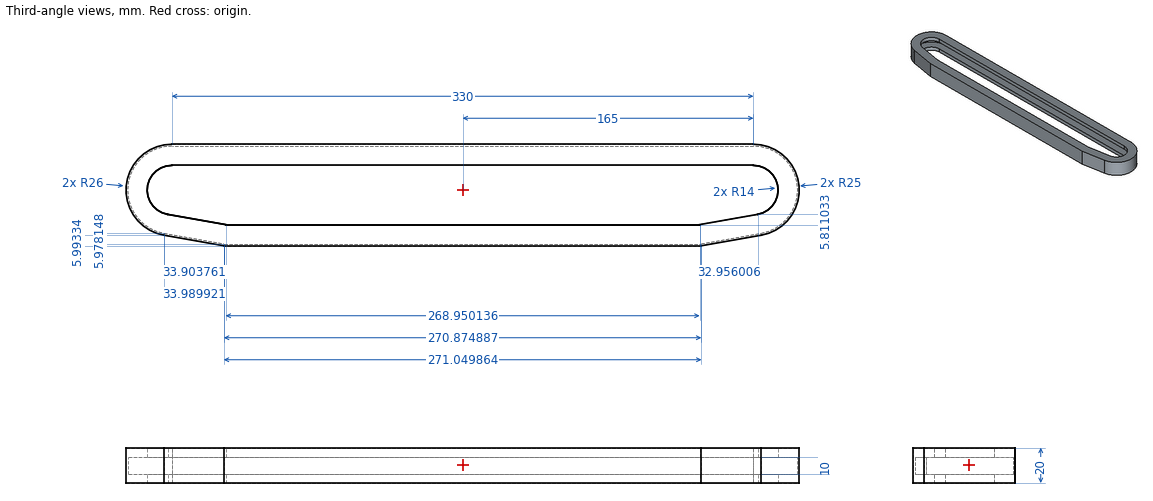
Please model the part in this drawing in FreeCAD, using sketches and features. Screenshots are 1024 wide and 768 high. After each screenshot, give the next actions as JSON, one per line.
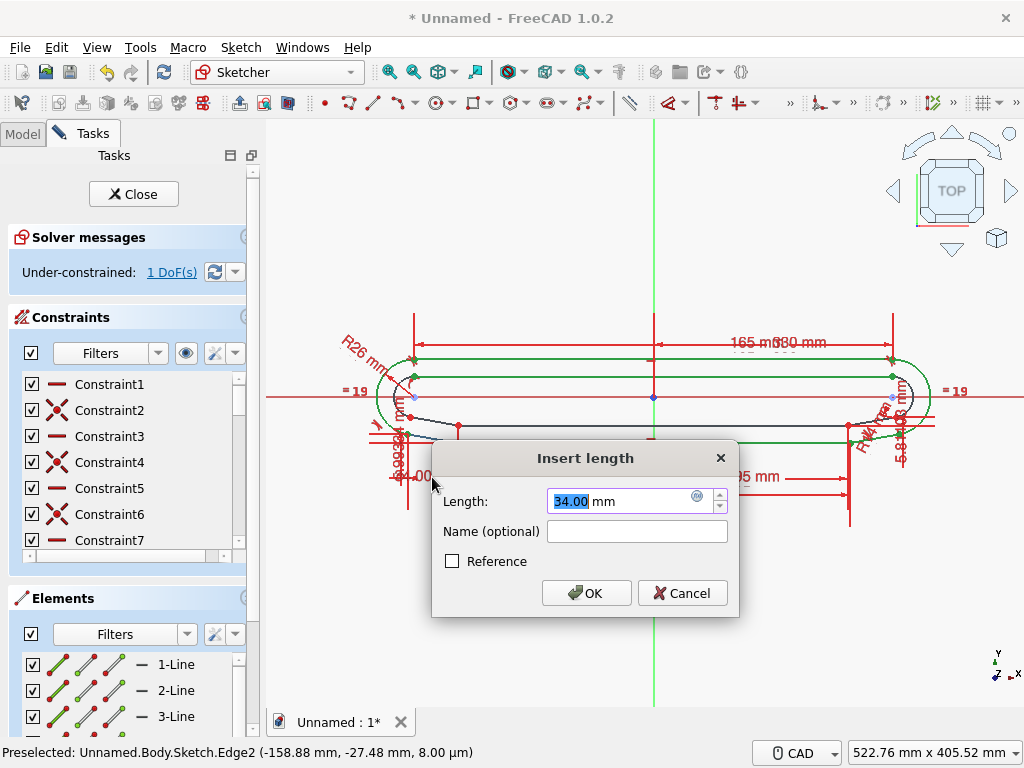
{"action": "type", "text": "33.989921"}
{"action": "key", "text": "Return"}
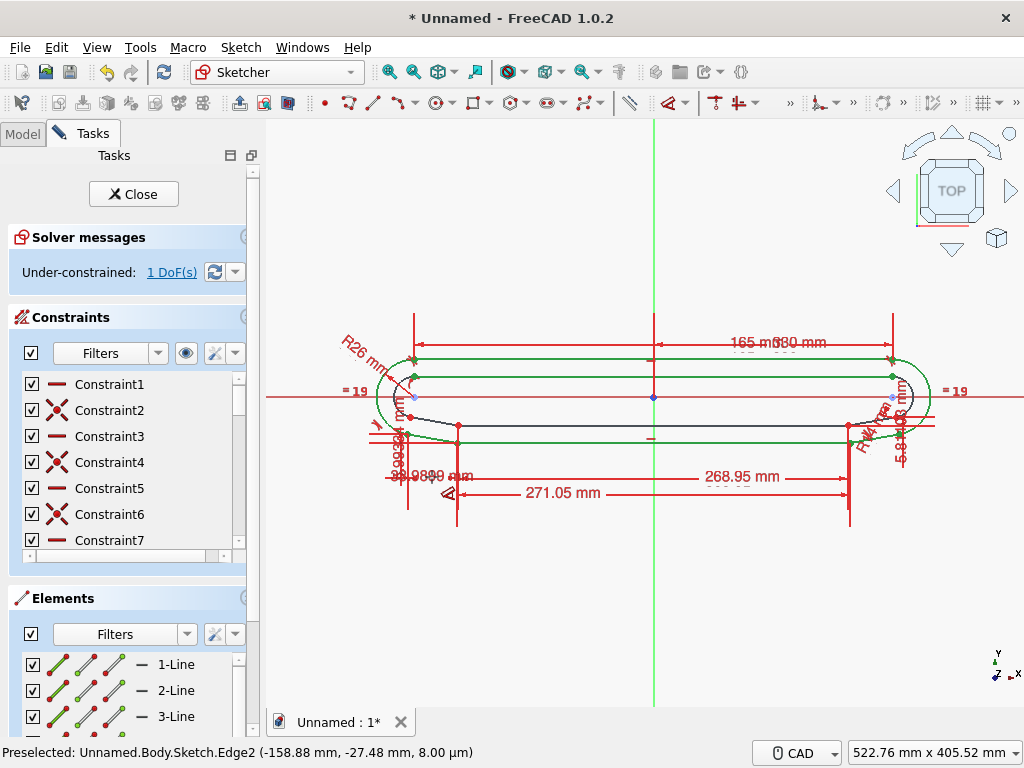
{"action": "scroll", "coordinate": [858, 424], "scroll_direction": "up", "scroll_amount": 2}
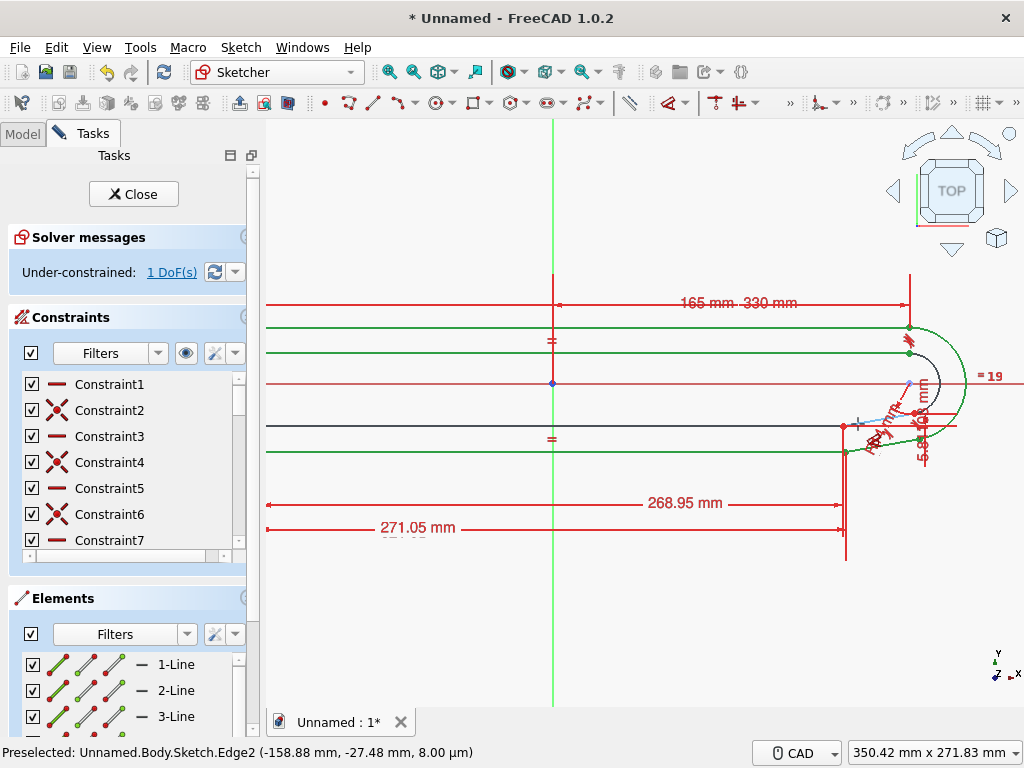
{"action": "left_click", "coordinate": [858, 424]}
{"action": "left_click", "coordinate": [851, 484]}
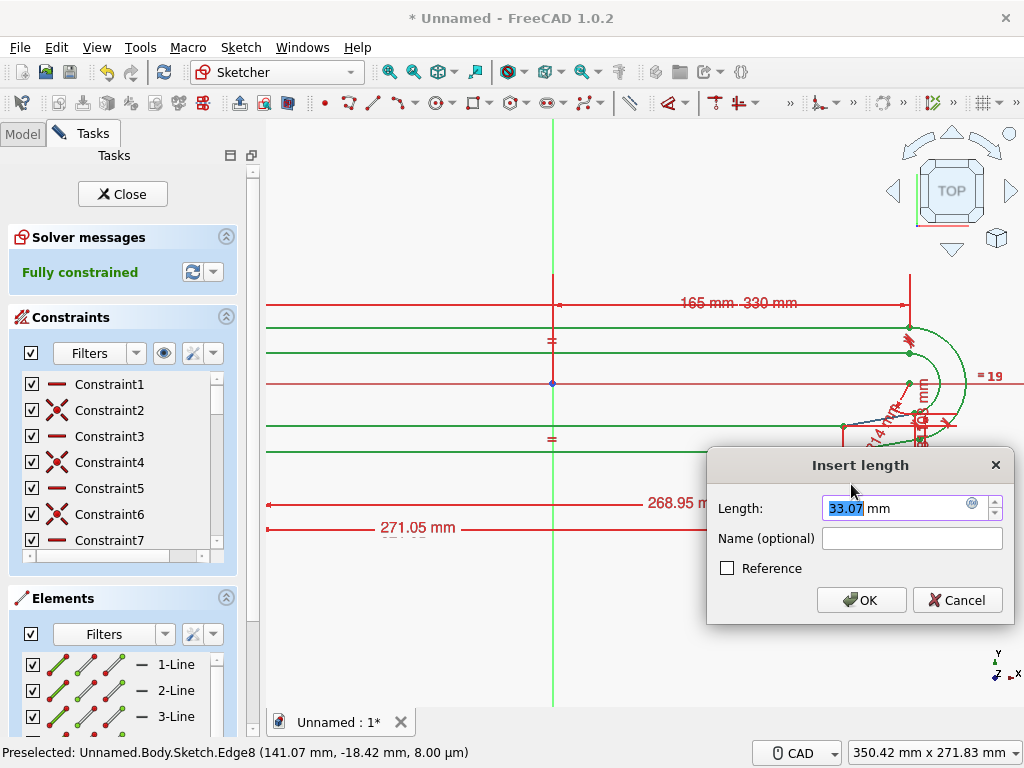
{"action": "type", "text": "32.956006"}
{"action": "key", "text": "Return"}
{"action": "key", "text": "Escape"}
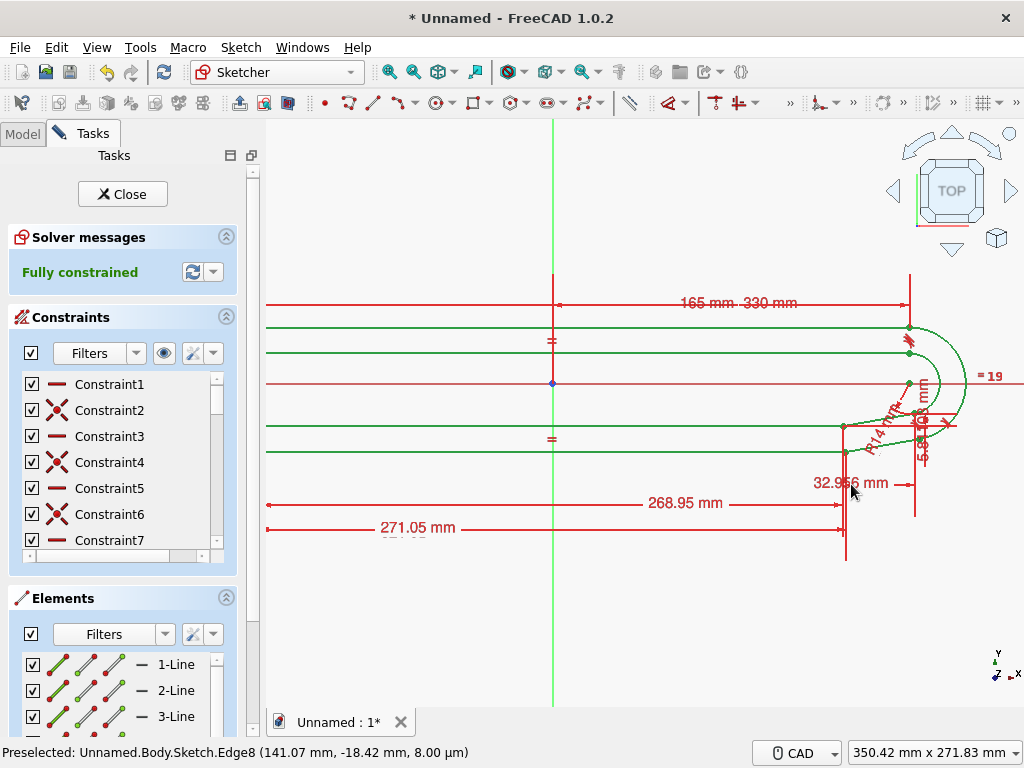
{"action": "left_click", "coordinate": [123, 194]}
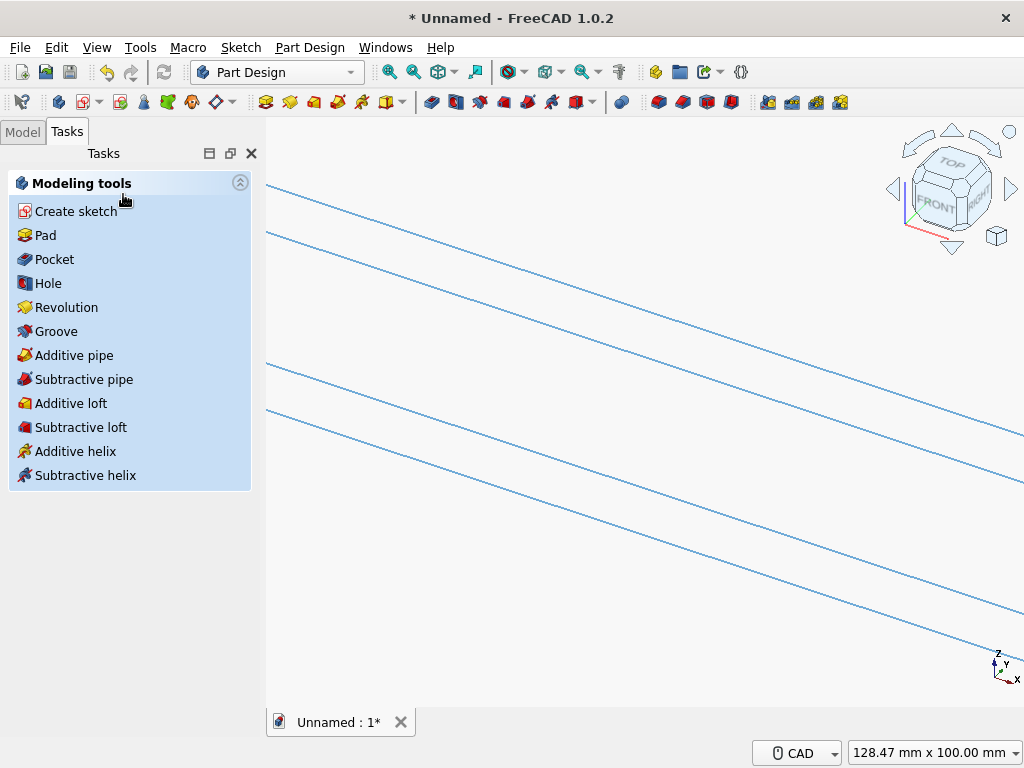
{"action": "left_click", "coordinate": [266, 102]}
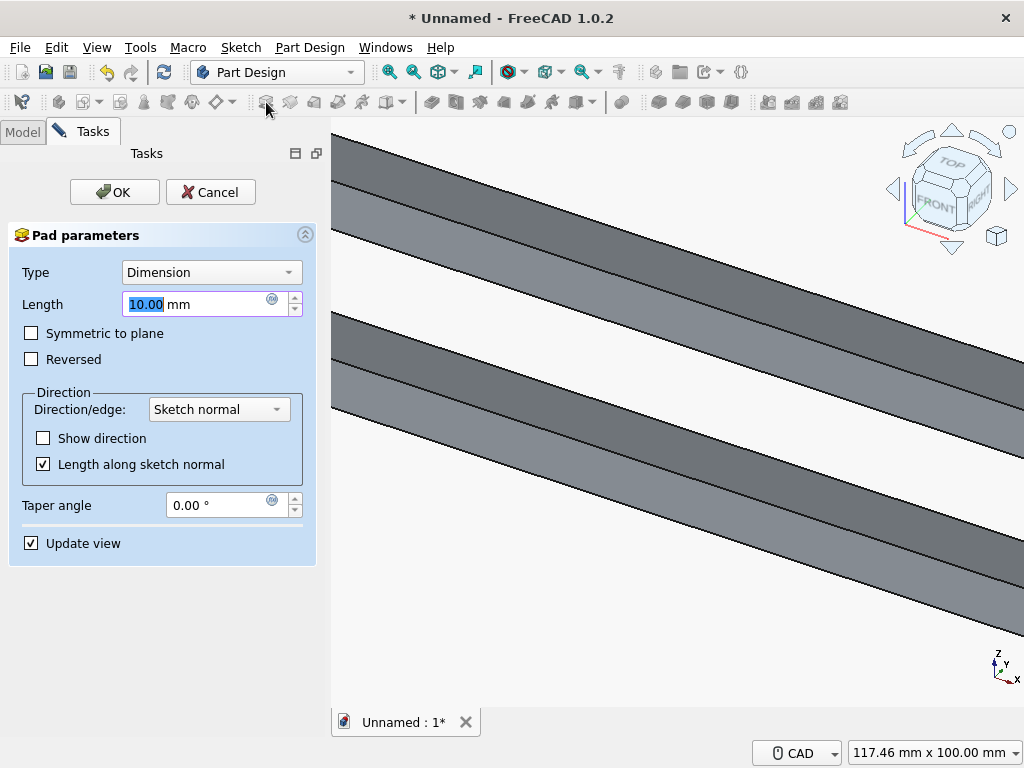
{"action": "type", "text": "20"}
{"action": "key", "text": "Tab"}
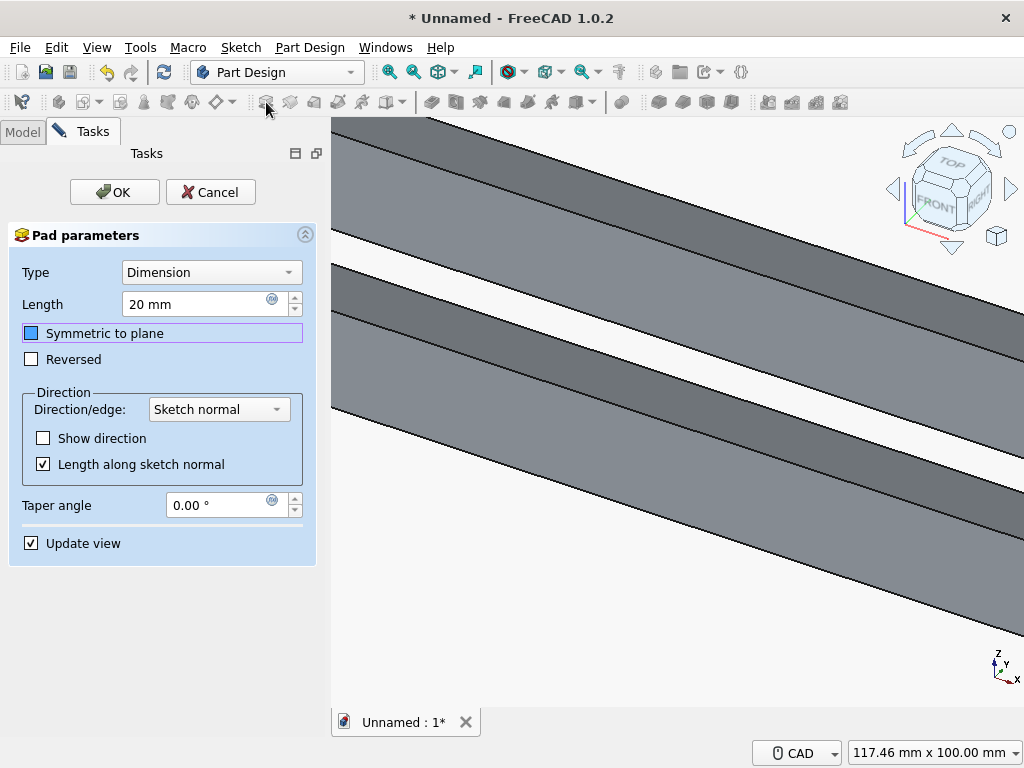
{"action": "left_click", "coordinate": [30, 333]}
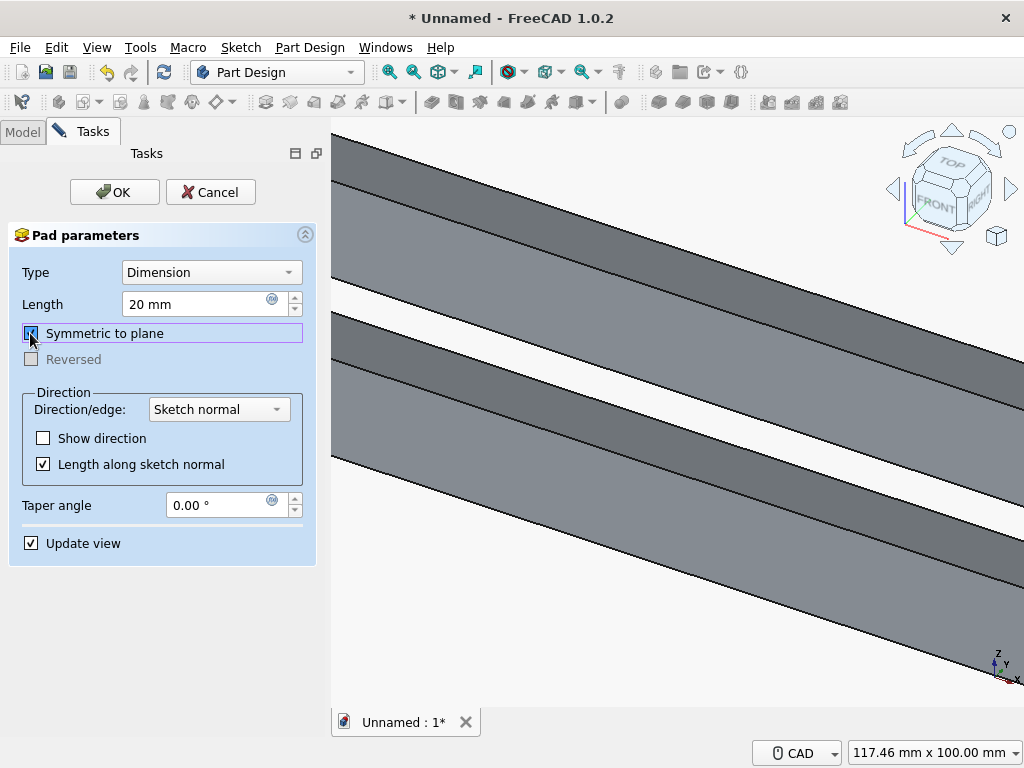
{"action": "left_click", "coordinate": [115, 192]}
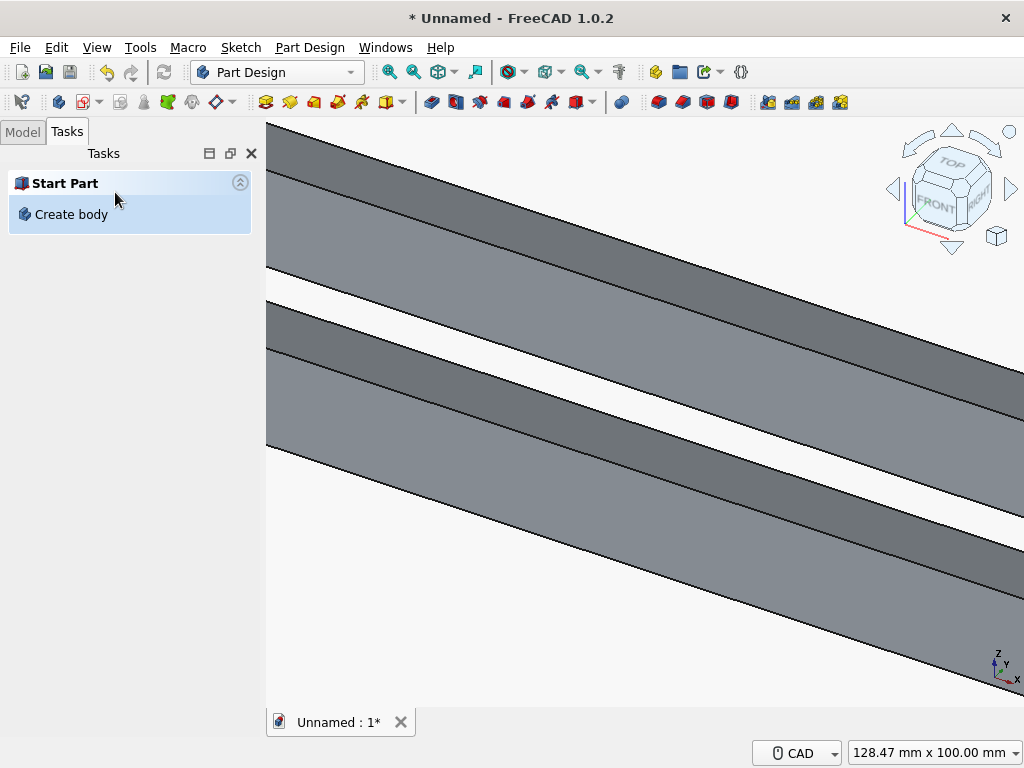
{"action": "left_click", "coordinate": [390, 72]}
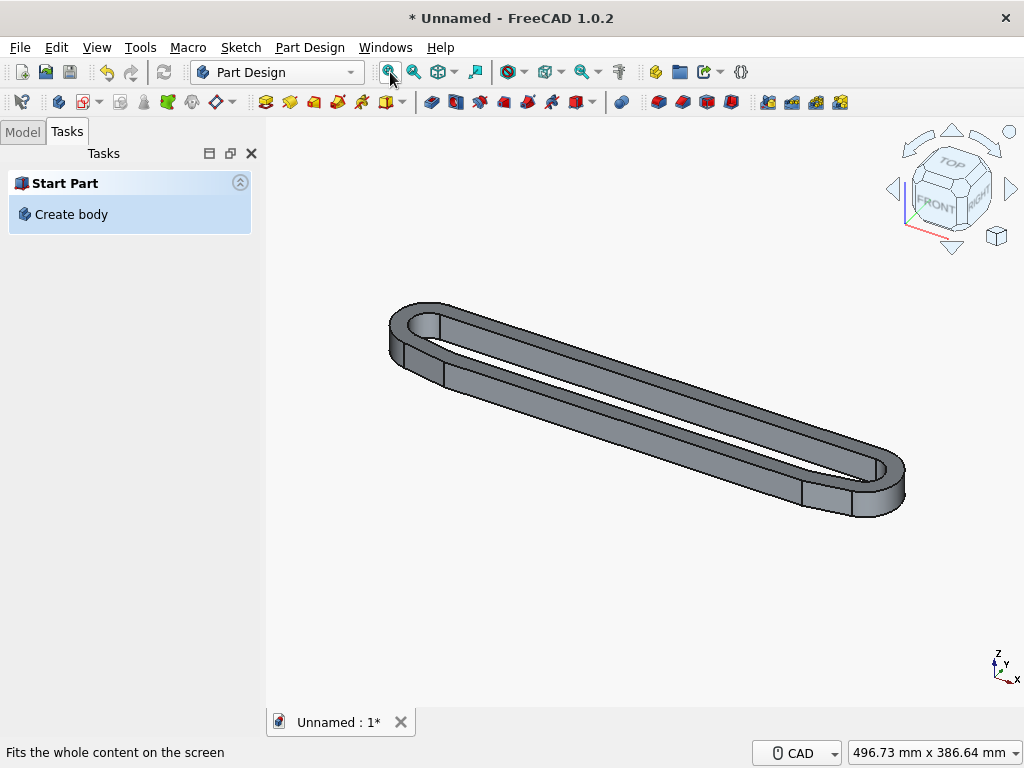
{"action": "left_click", "coordinate": [84, 102]}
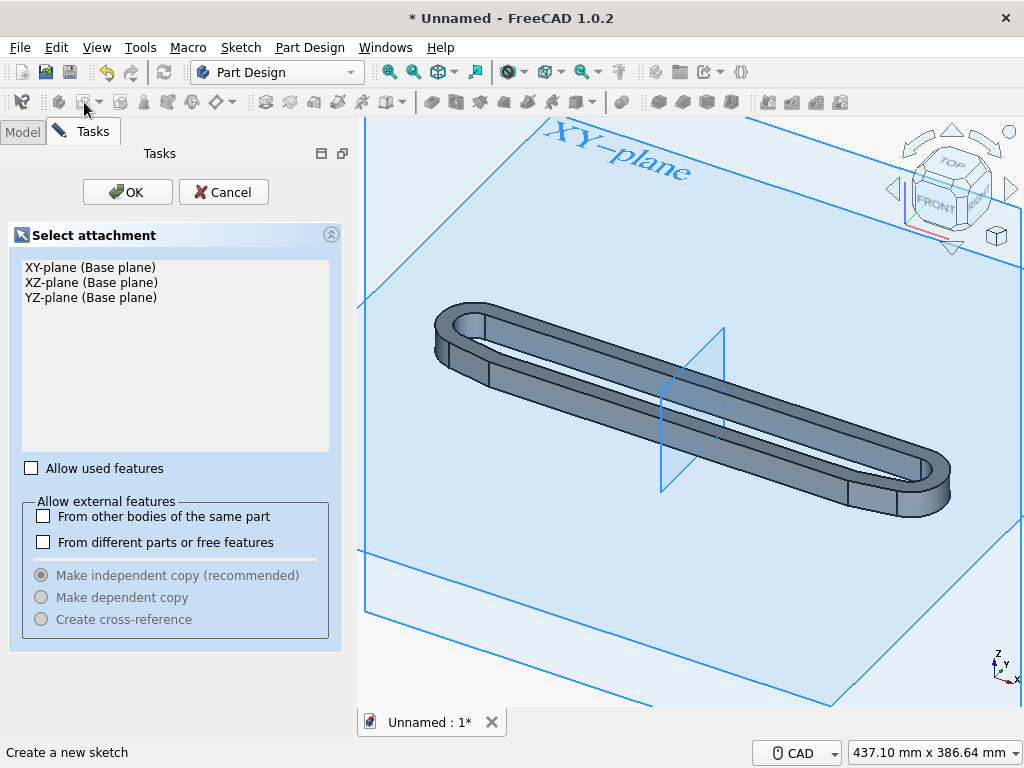
{"action": "left_click", "coordinate": [82, 268]}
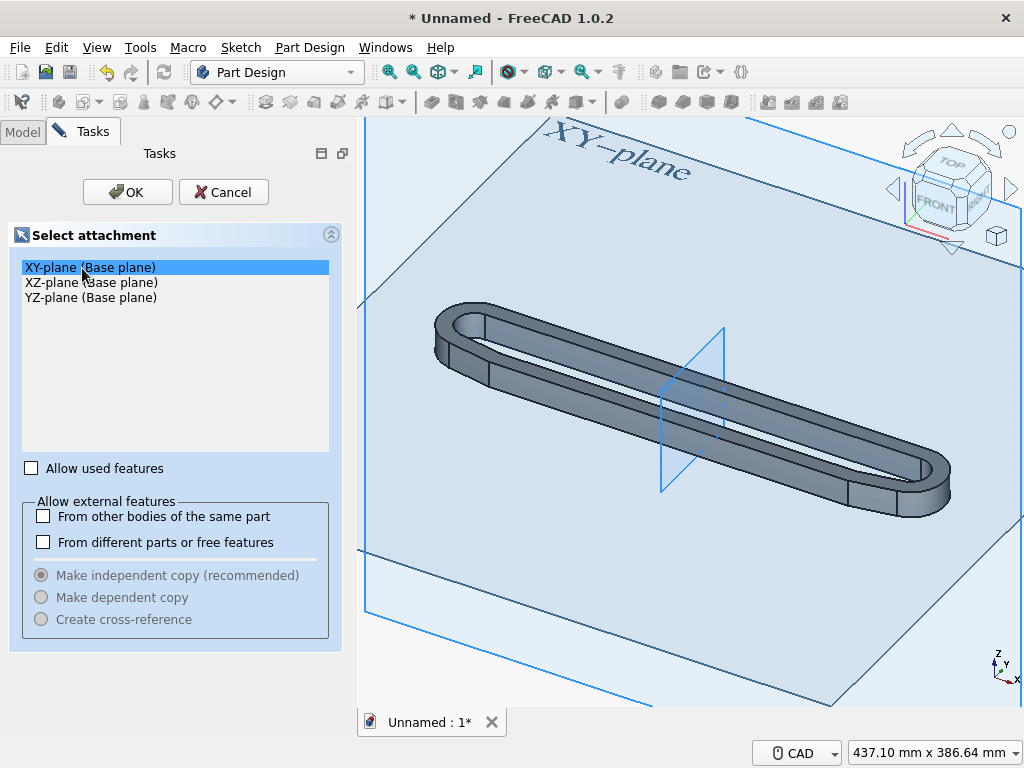
{"action": "left_click", "coordinate": [128, 192]}